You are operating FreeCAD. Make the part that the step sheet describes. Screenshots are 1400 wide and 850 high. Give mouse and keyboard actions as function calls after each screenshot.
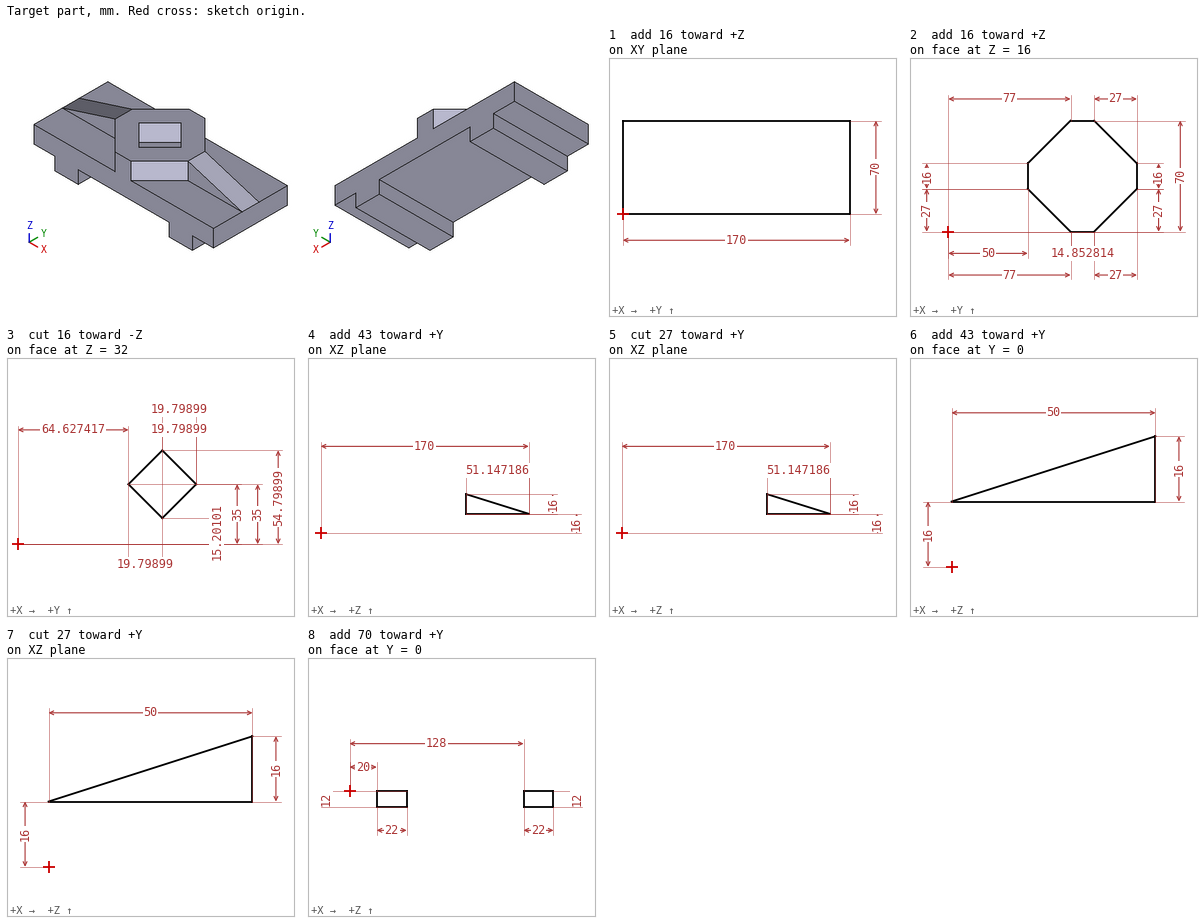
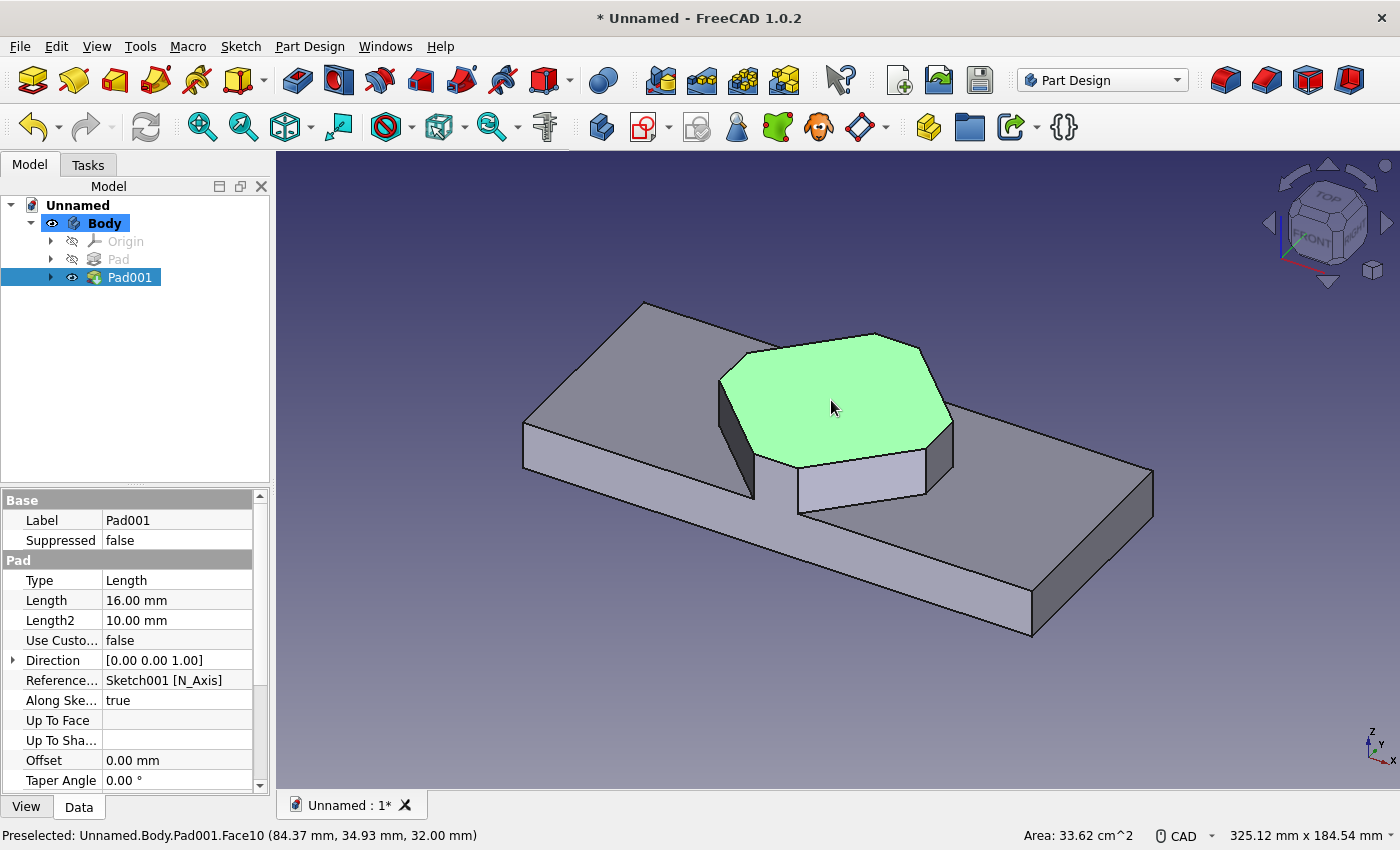
click(642, 128)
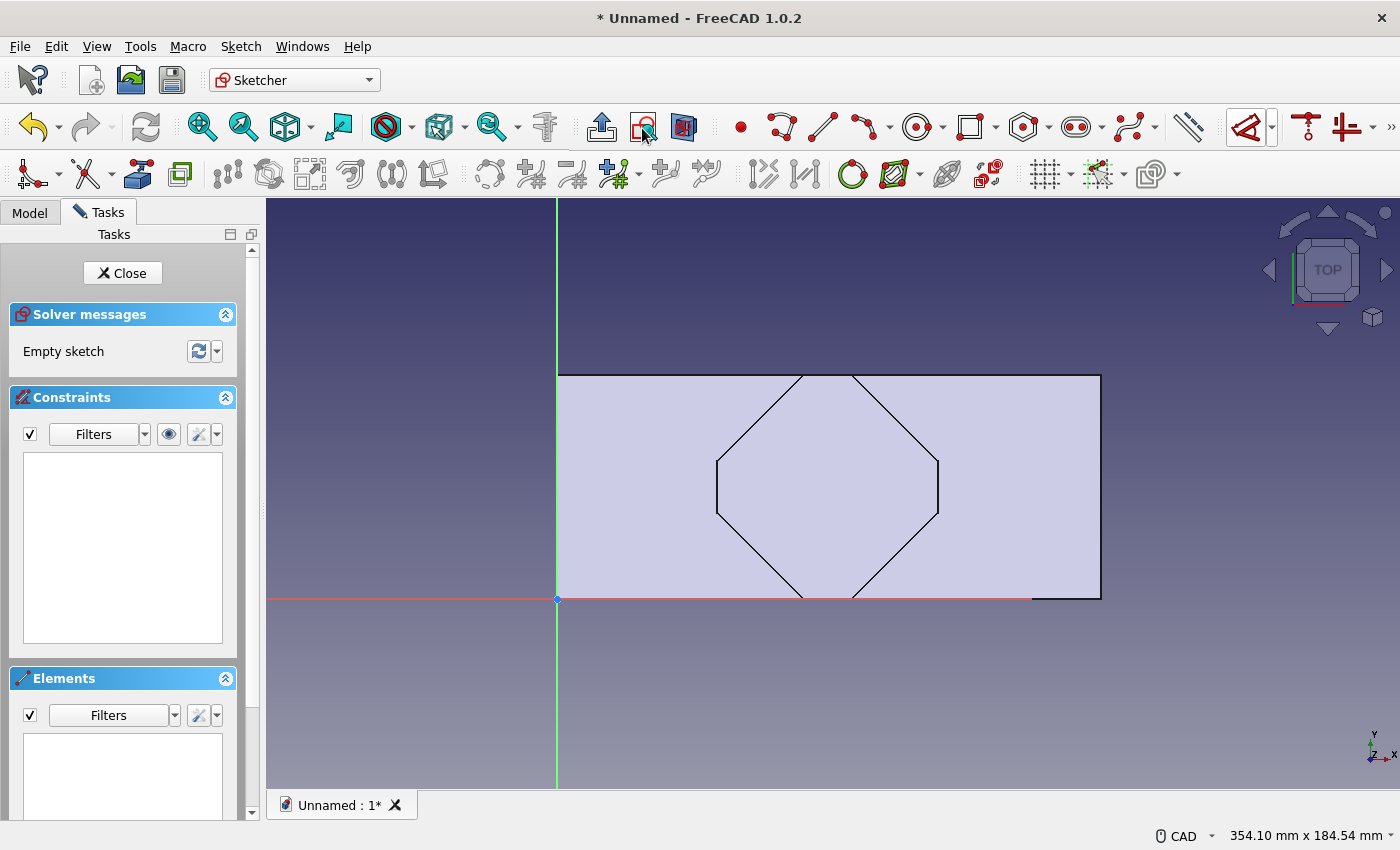
scroll(864, 483, up, 5)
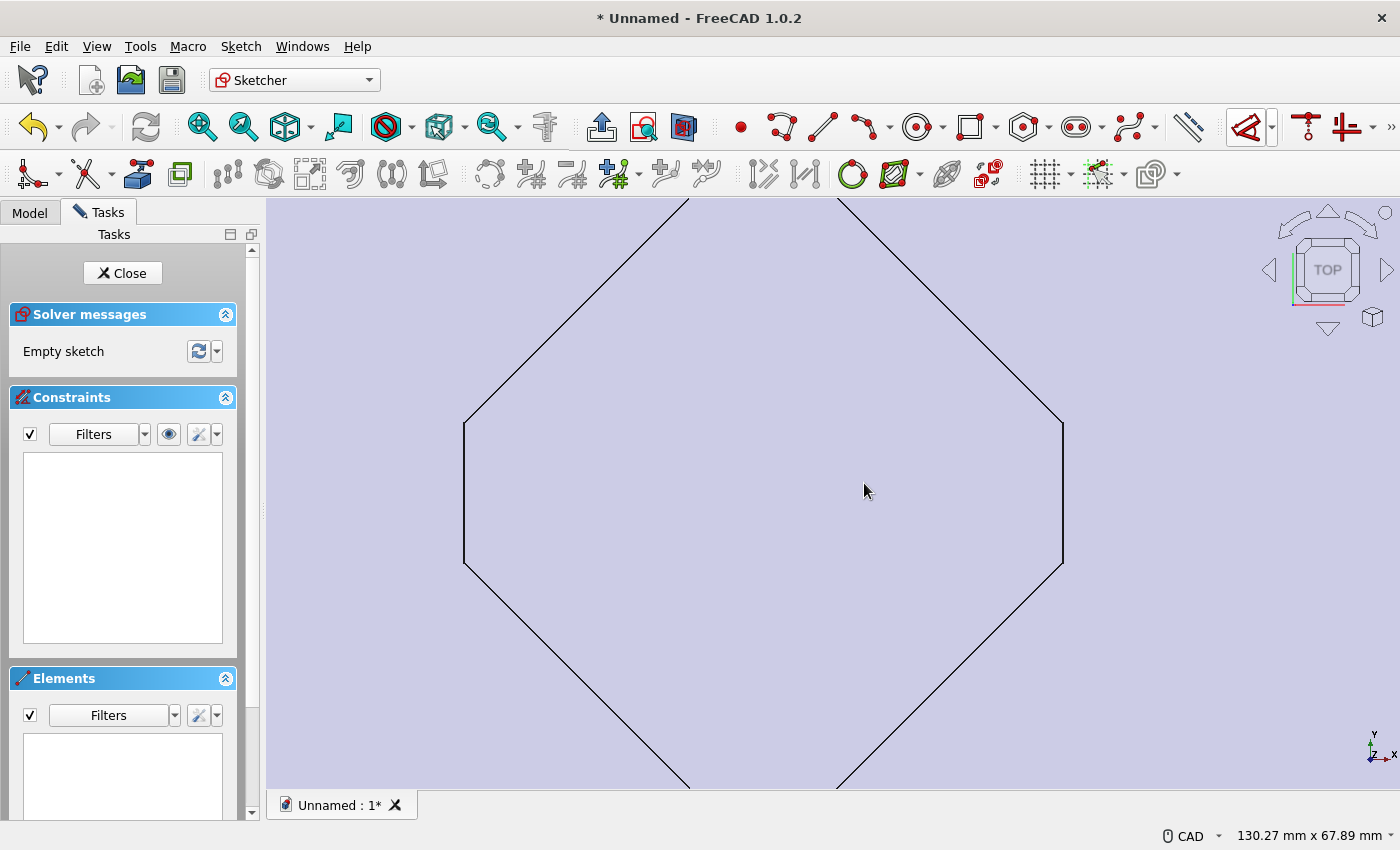
key(g)
key(m)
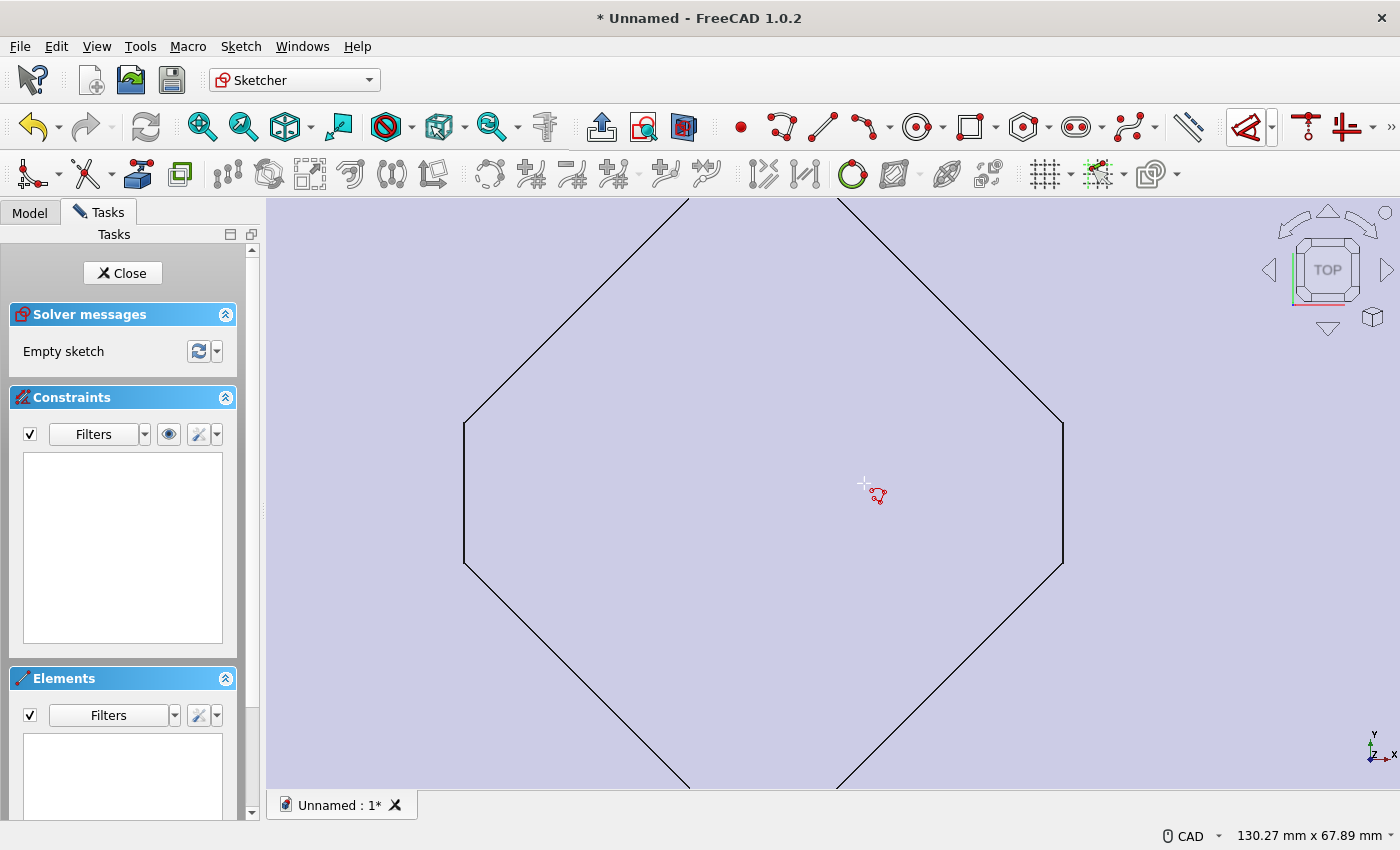
click(591, 493)
click(764, 665)
click(936, 493)
click(764, 321)
click(591, 494)
key(Escape)
key(Escape)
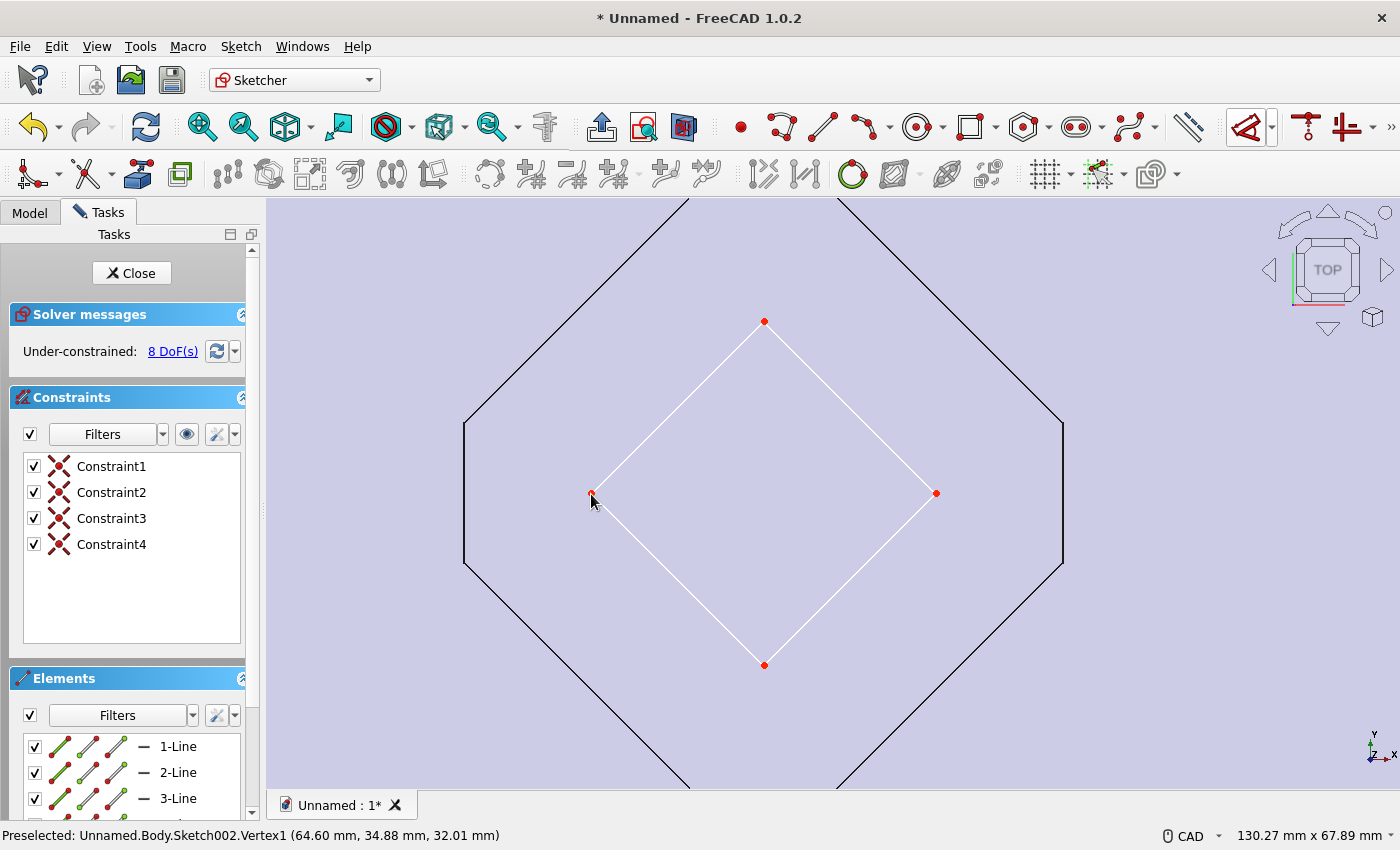
key(d)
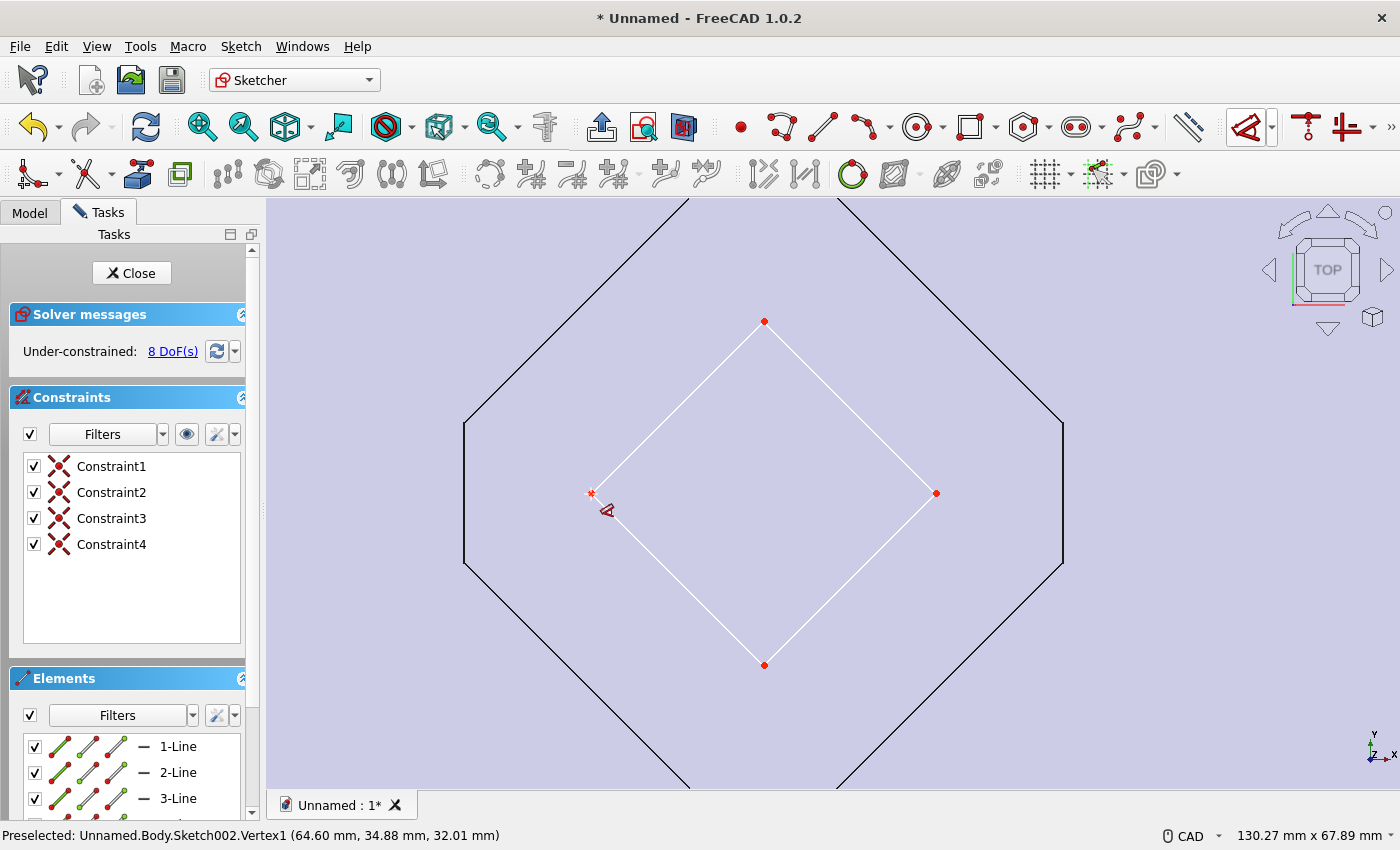
click(591, 494)
click(625, 628)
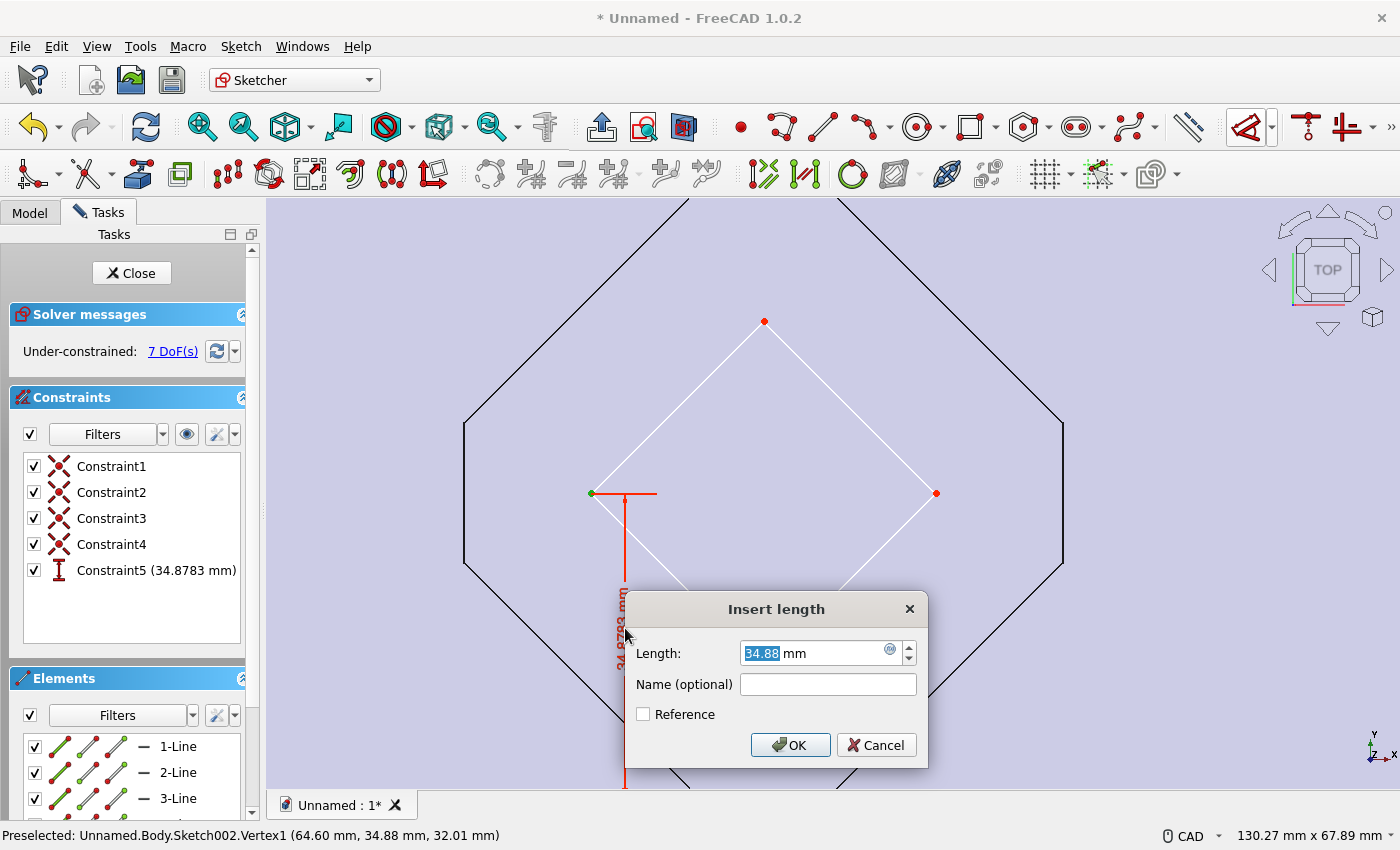
text(35)
key(Return)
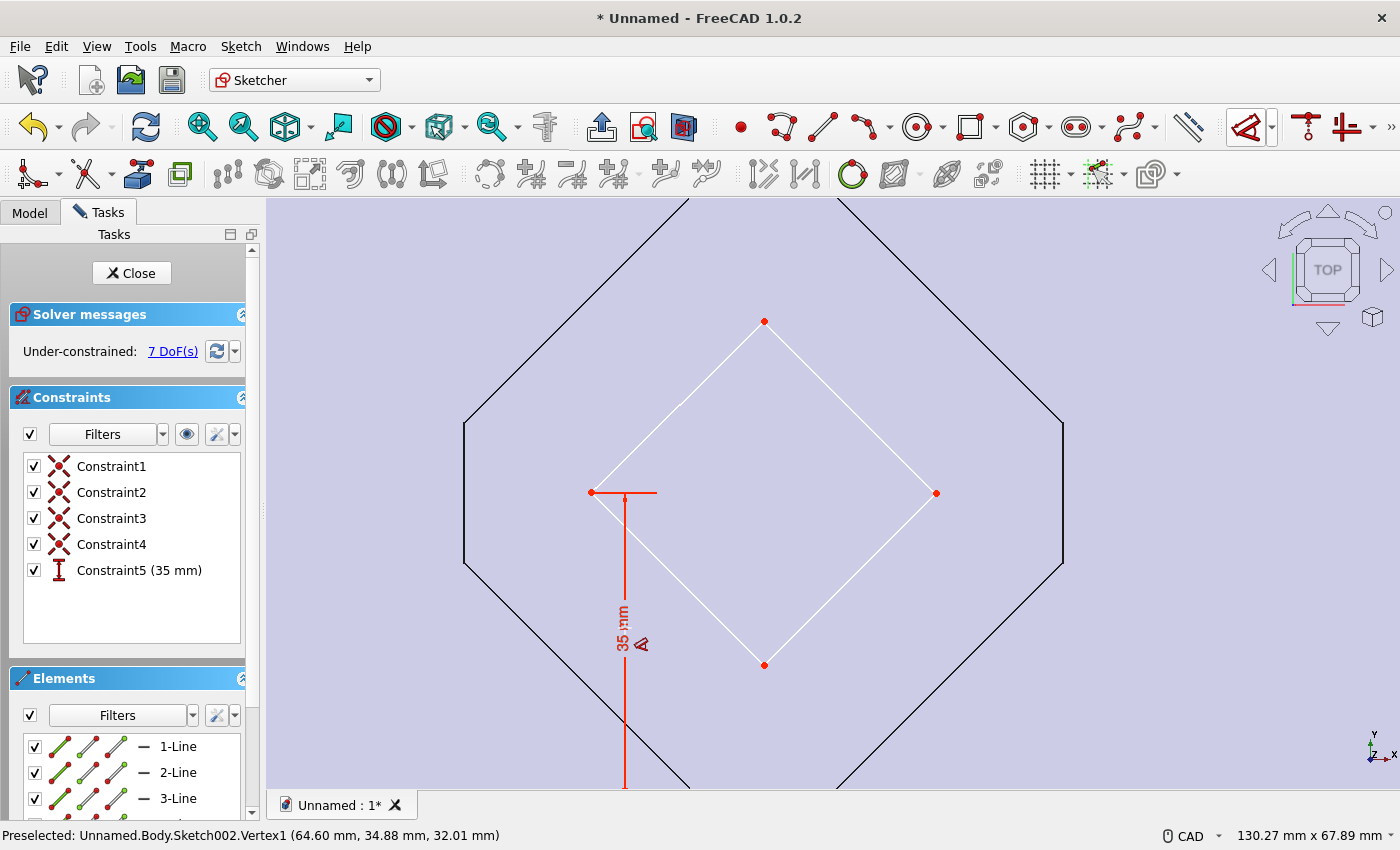
click(936, 494)
click(970, 628)